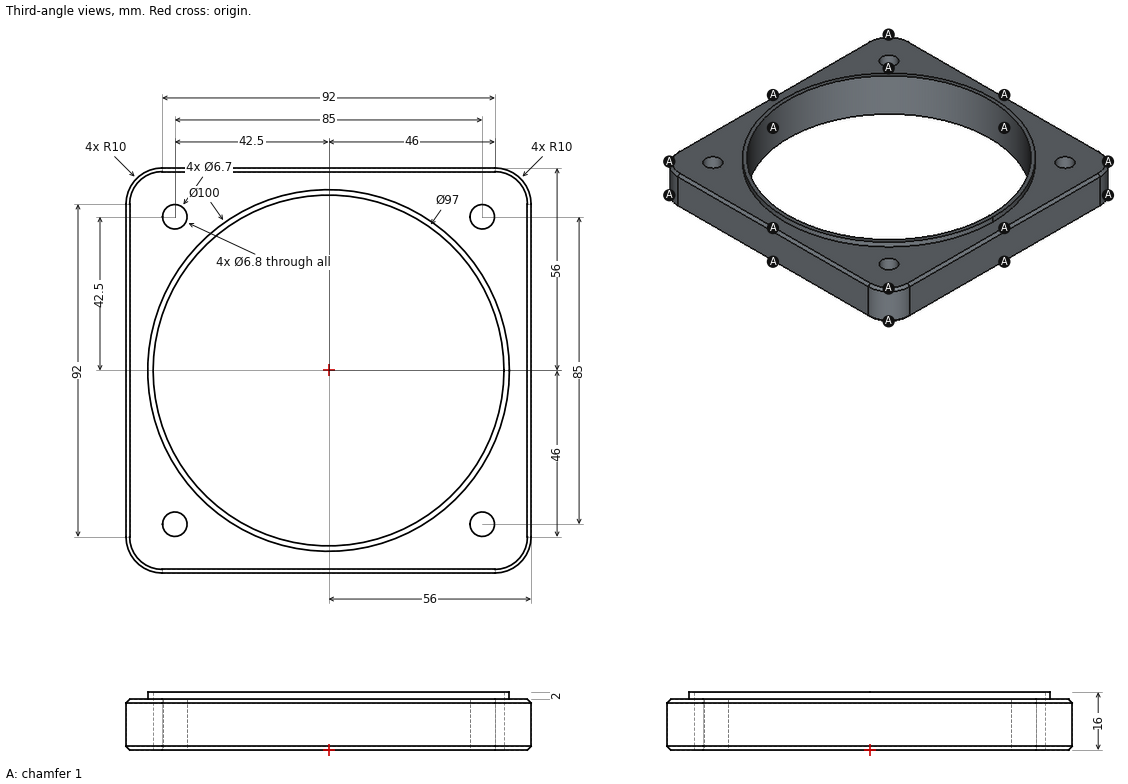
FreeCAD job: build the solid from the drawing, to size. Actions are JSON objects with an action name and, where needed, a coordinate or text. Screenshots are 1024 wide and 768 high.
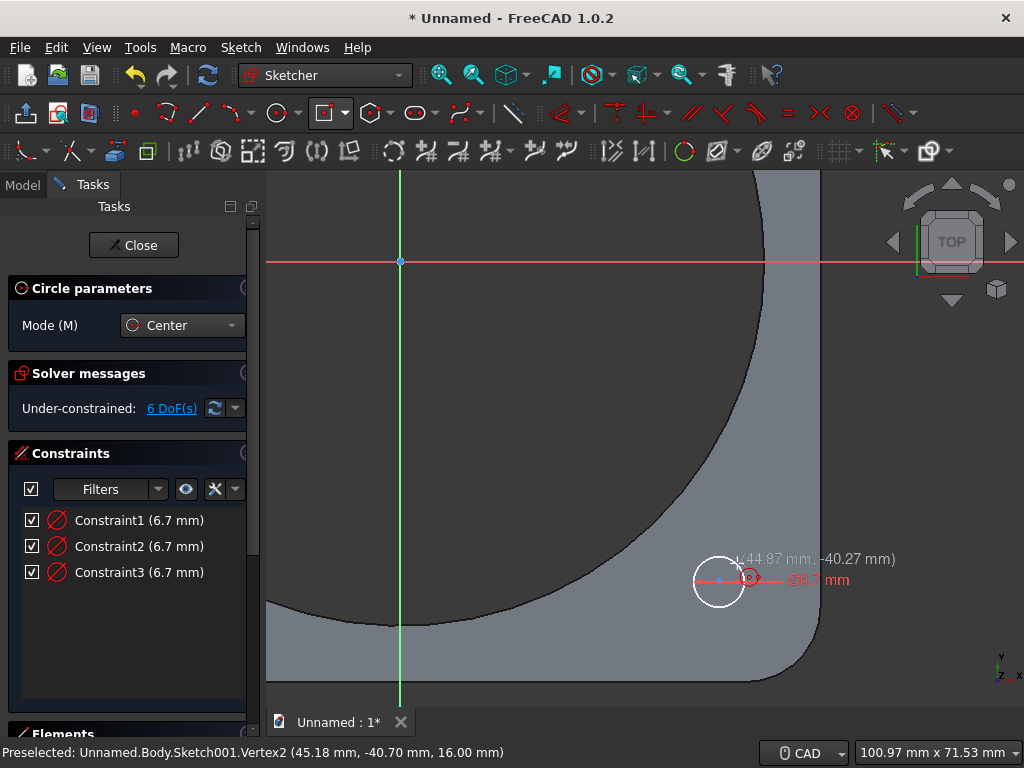
{"action": "scroll", "coordinate": [720, 583], "scroll_direction": "down", "scroll_amount": 4}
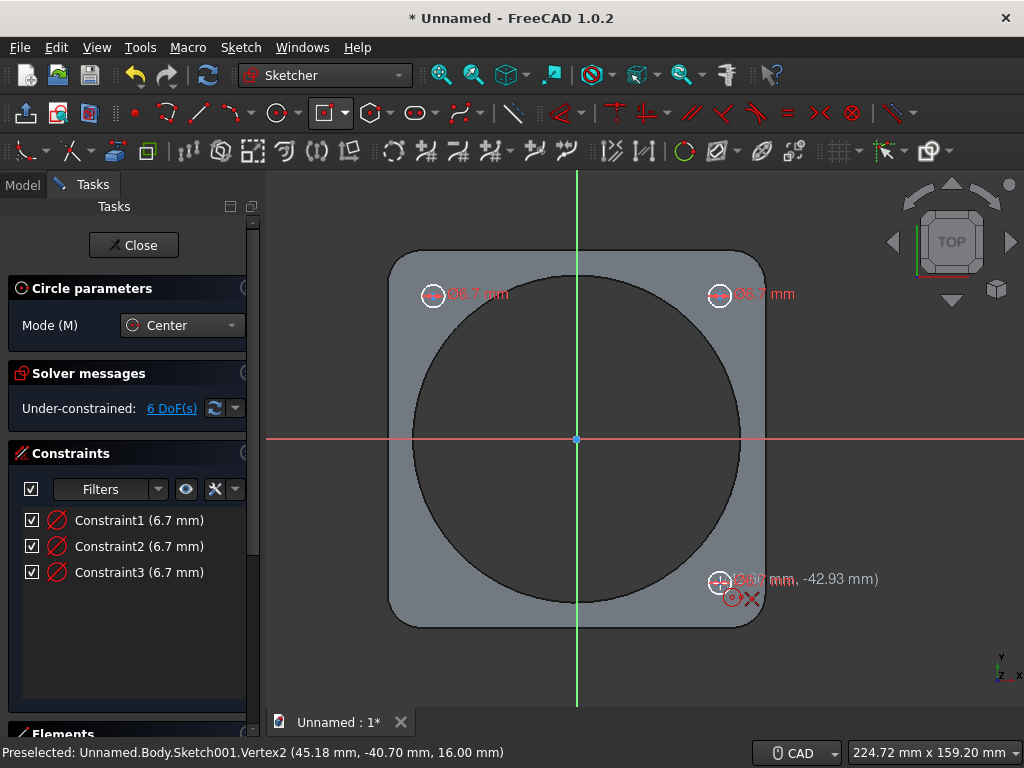
{"action": "scroll", "coordinate": [433, 582], "scroll_direction": "up", "scroll_amount": 4}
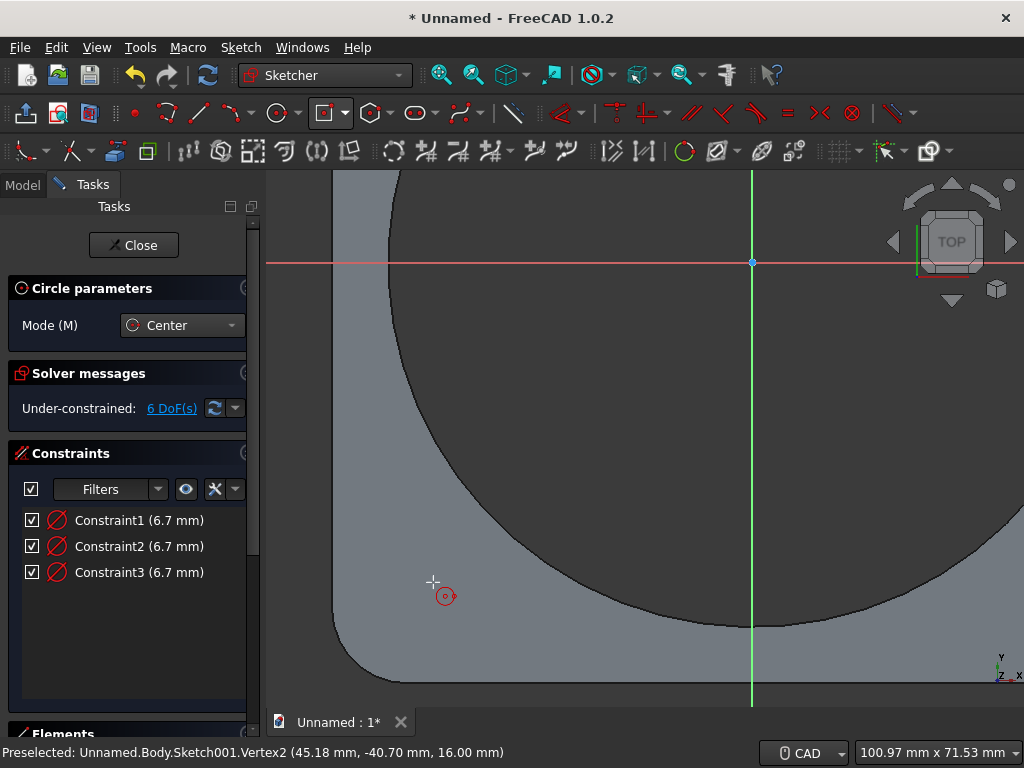
{"action": "left_click", "coordinate": [433, 582]}
{"action": "mouse_move", "coordinate": [451, 564]}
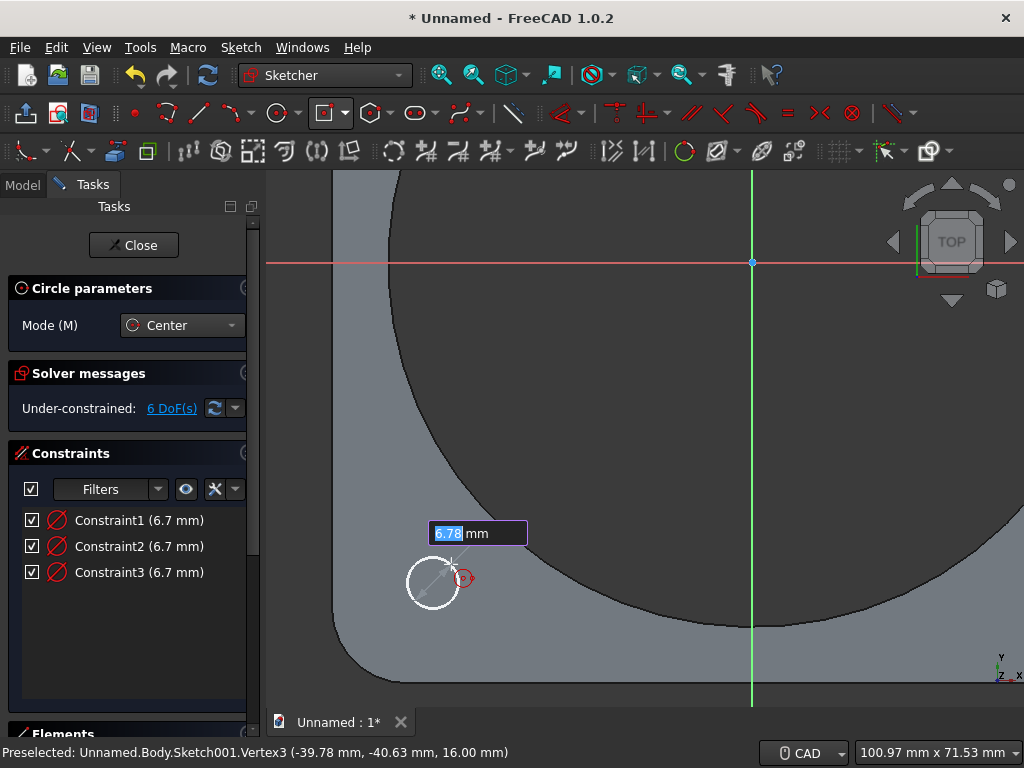
{"action": "type", "text": "6.7"}
{"action": "key", "text": "Return"}
{"action": "key", "text": "Escape"}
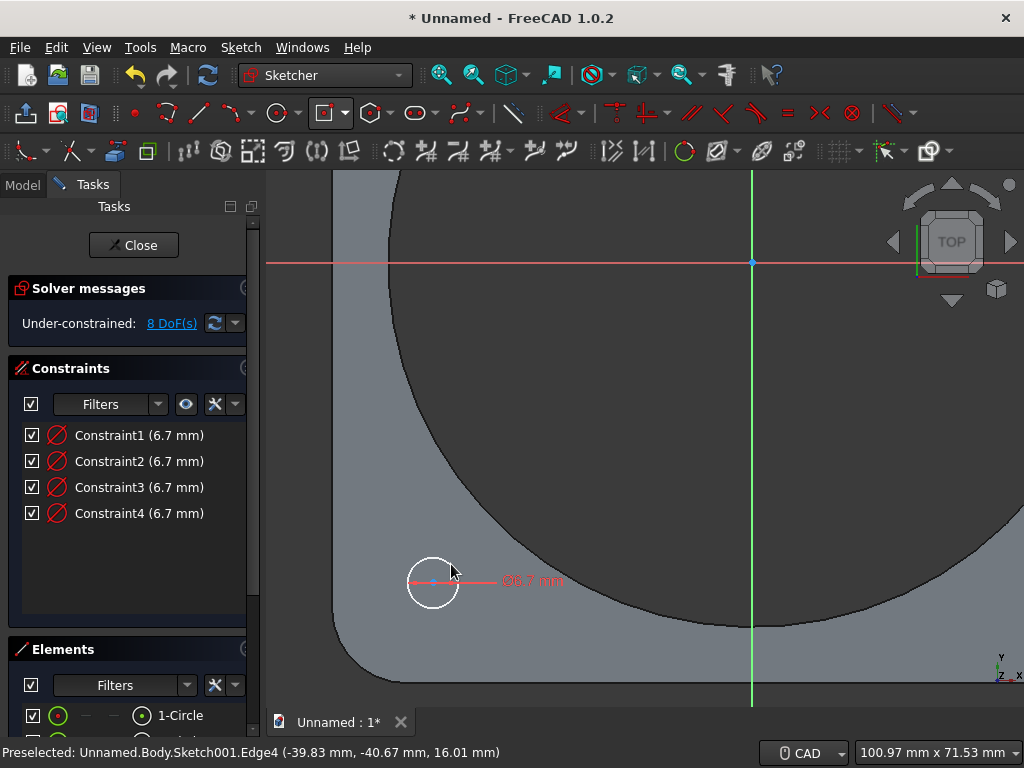
{"action": "scroll", "coordinate": [433, 582], "scroll_direction": "down", "scroll_amount": 4}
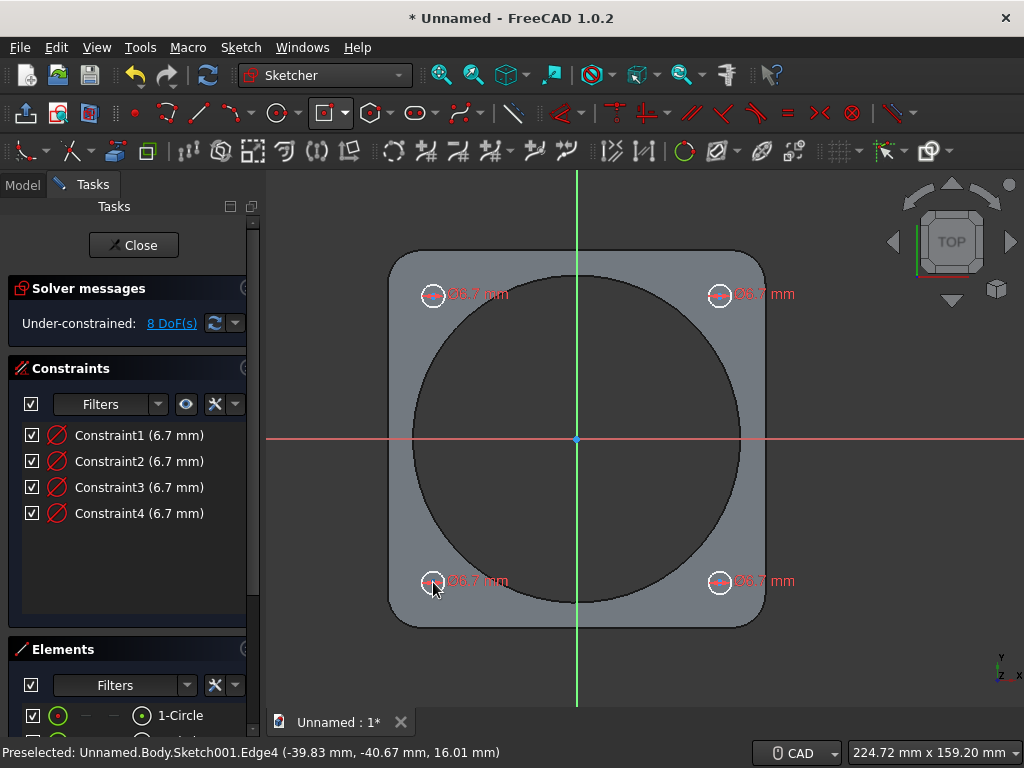
{"action": "left_click", "coordinate": [433, 296]}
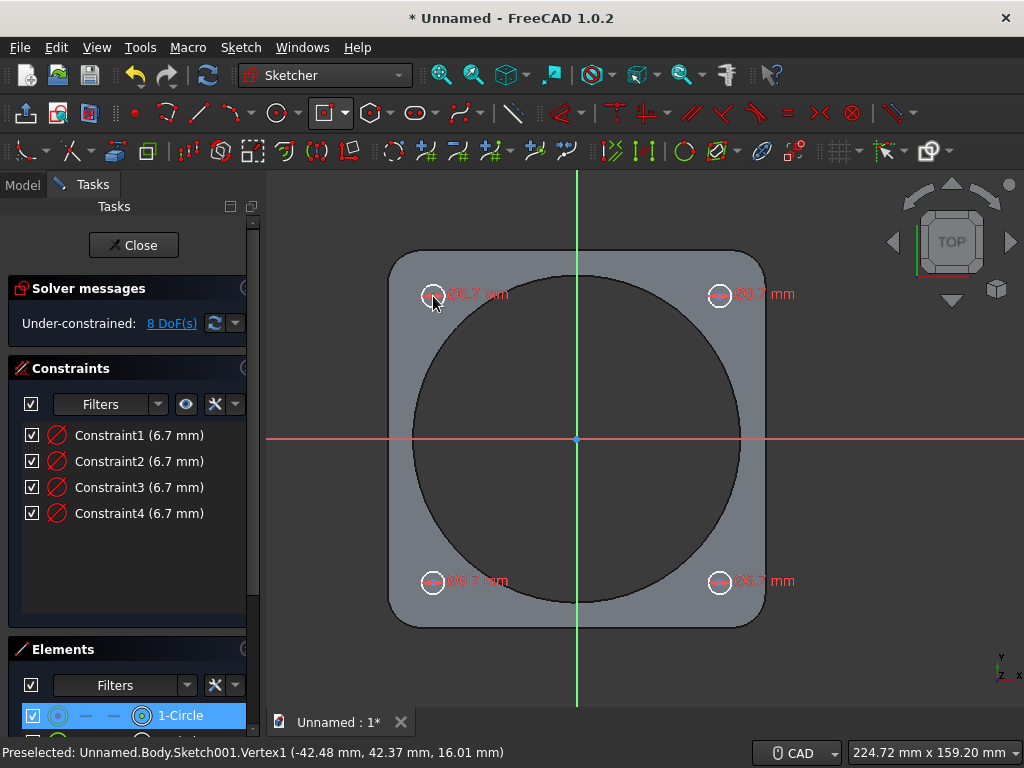
{"action": "left_click", "coordinate": [720, 296]}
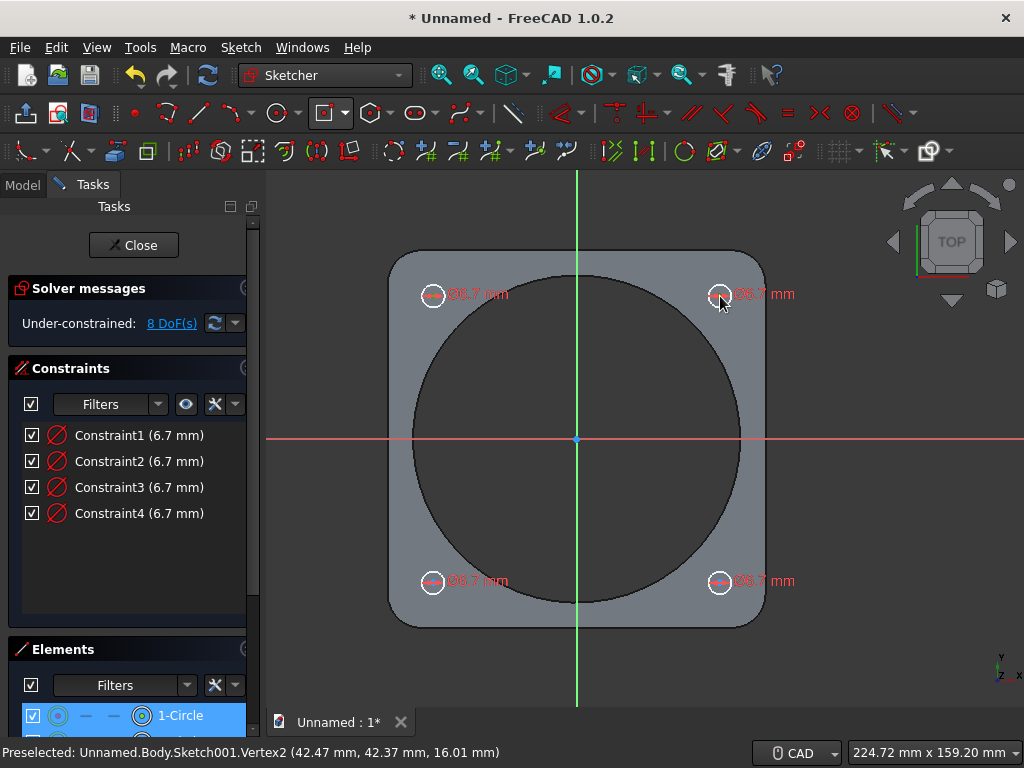
{"action": "left_click", "coordinate": [670, 114]}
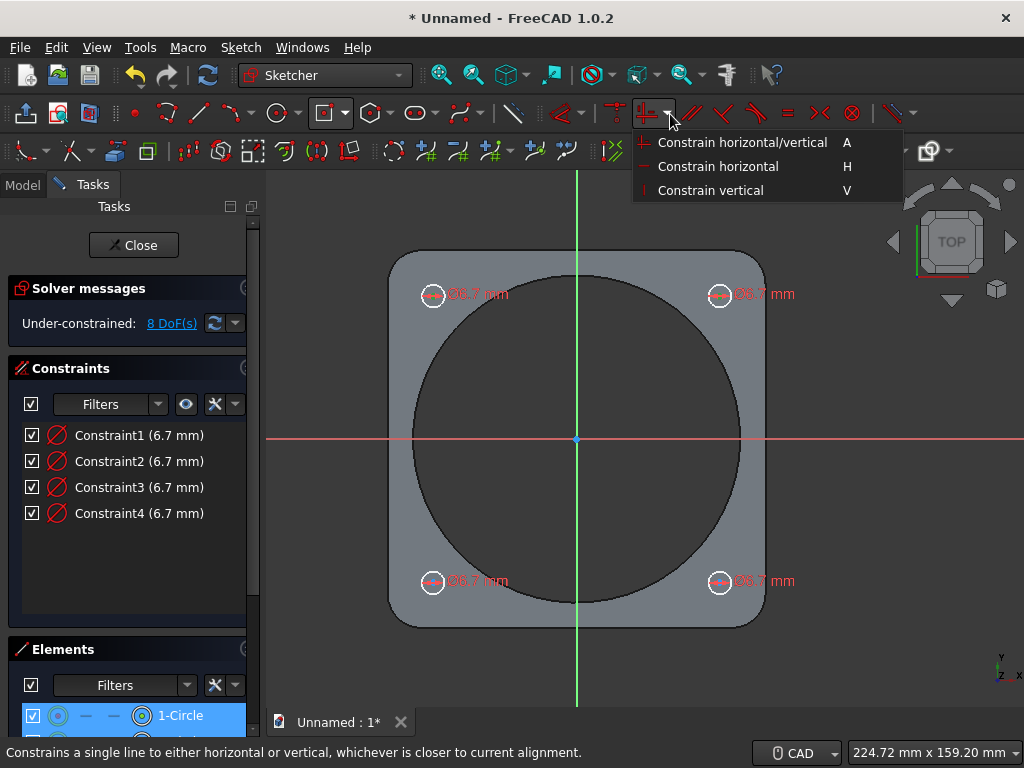
{"action": "left_click", "coordinate": [768, 166]}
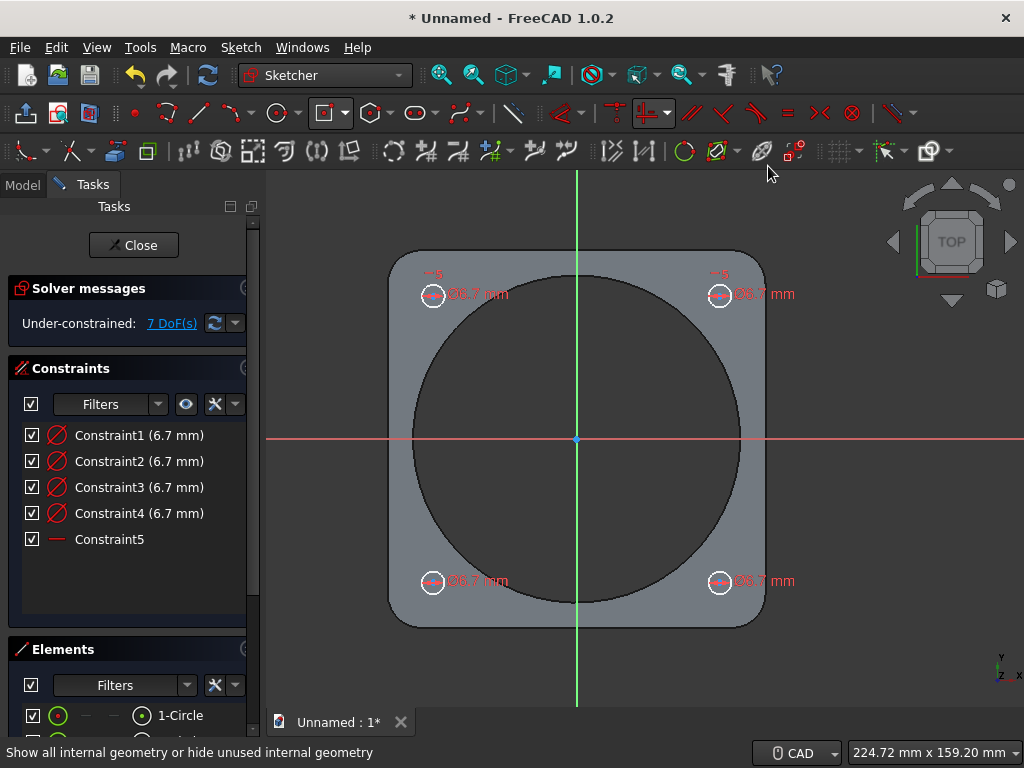
{"action": "left_click", "coordinate": [720, 296]}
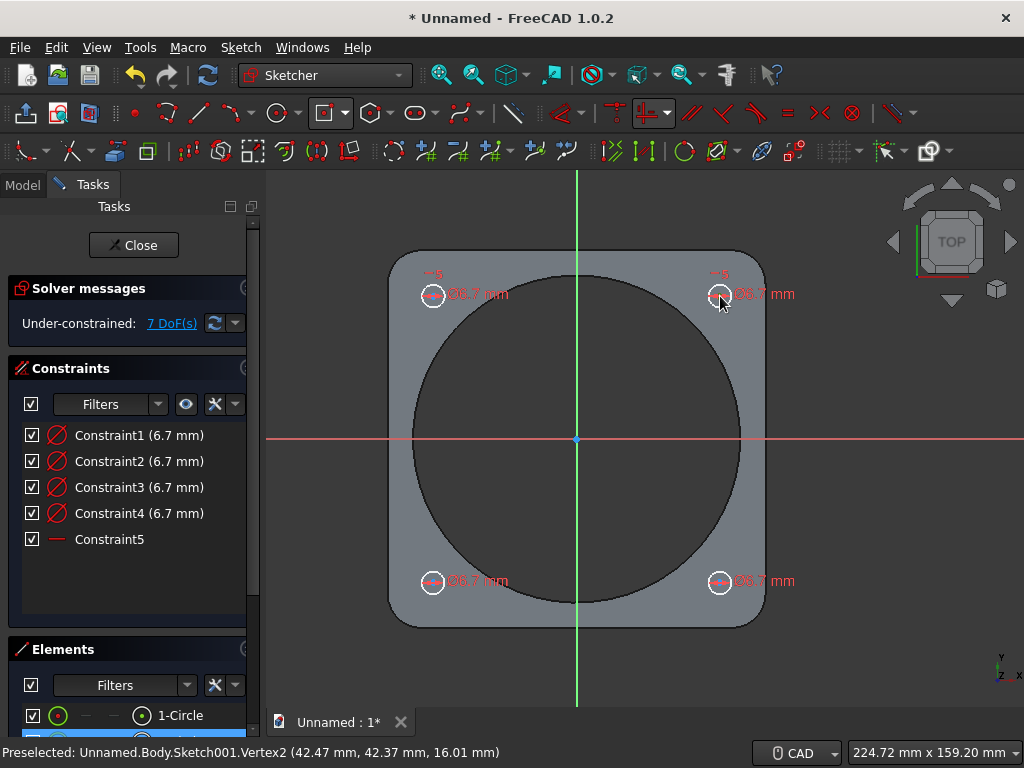
{"action": "left_click", "coordinate": [720, 583]}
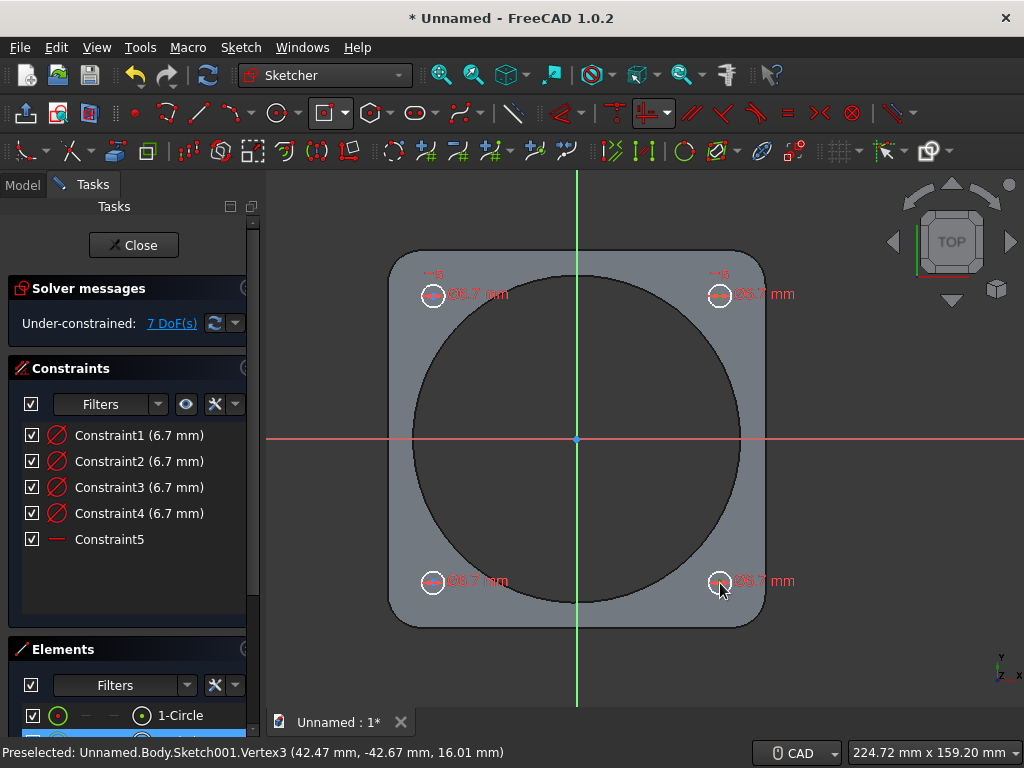
{"action": "left_click", "coordinate": [670, 114]}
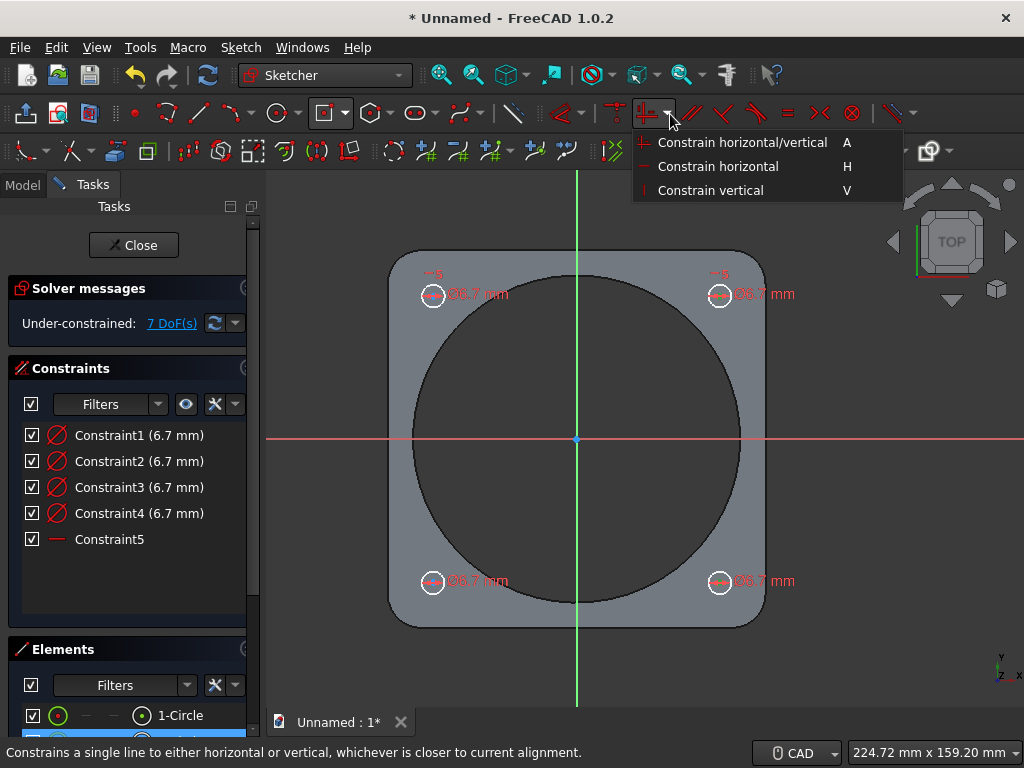
{"action": "left_click", "coordinate": [768, 190]}